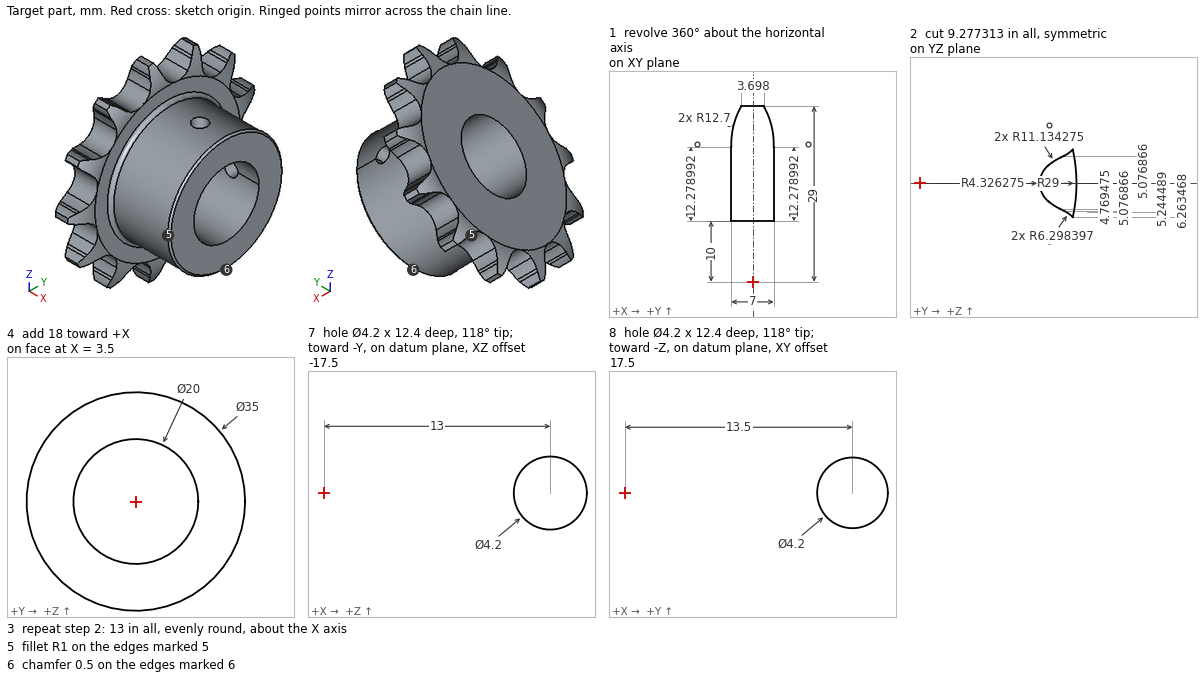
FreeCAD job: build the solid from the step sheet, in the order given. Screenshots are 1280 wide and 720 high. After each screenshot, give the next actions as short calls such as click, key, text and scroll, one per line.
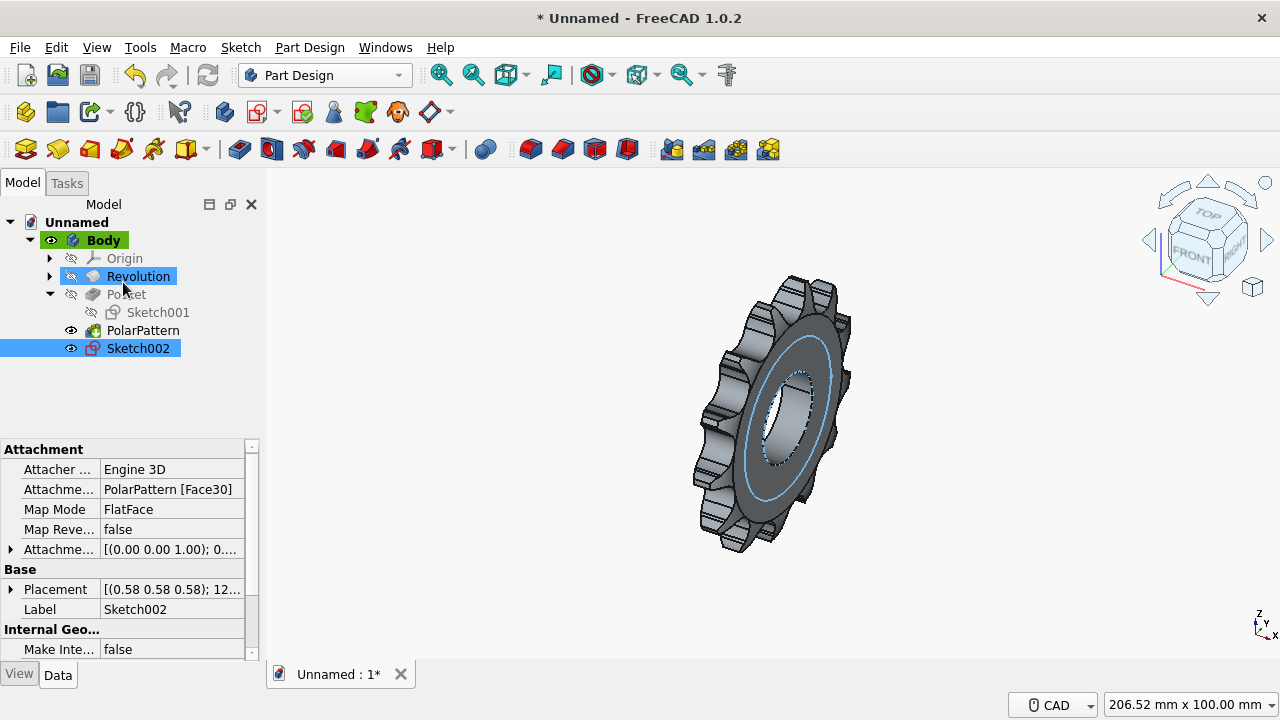
click(26, 150)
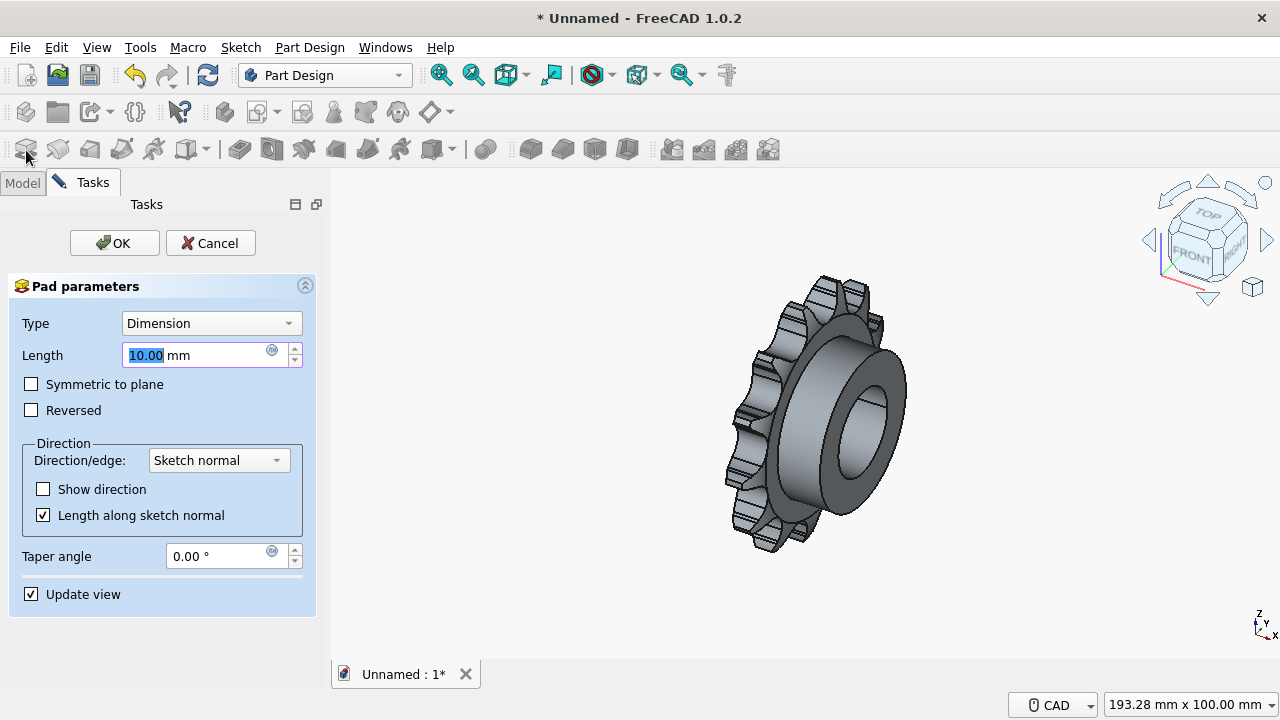
text(18)
key(Tab)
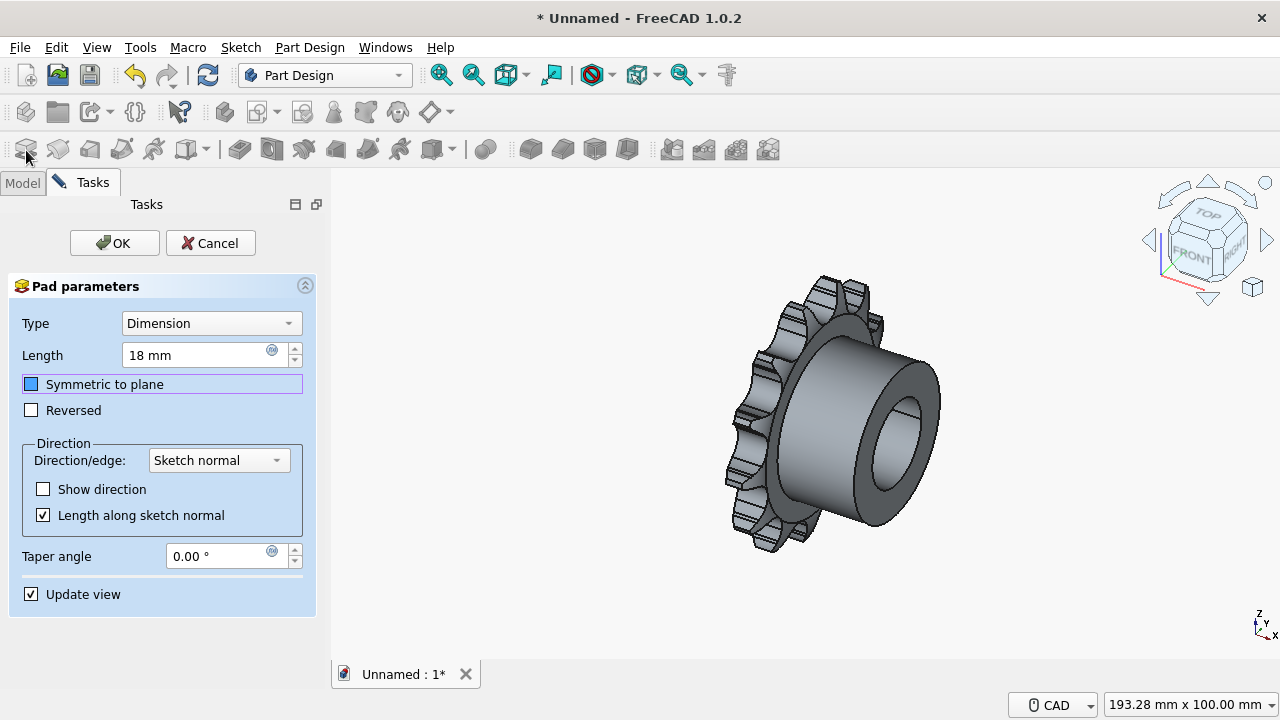
click(115, 243)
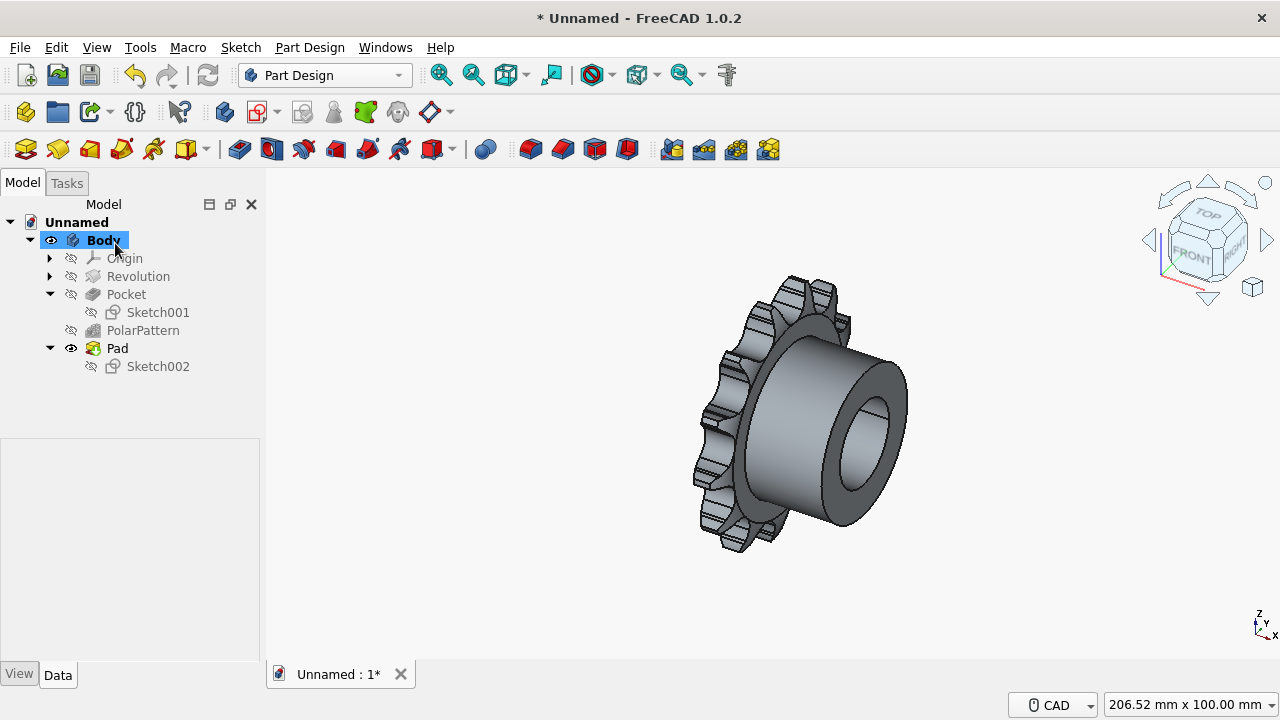
key(0)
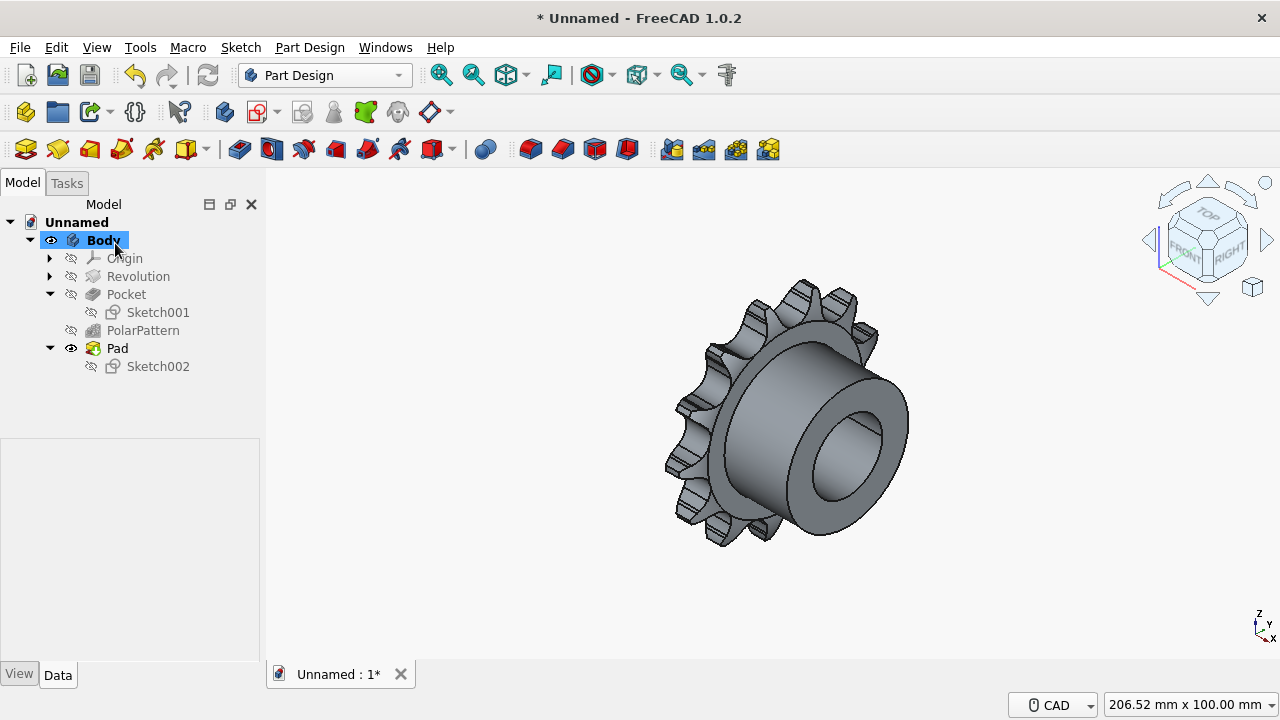
key(2)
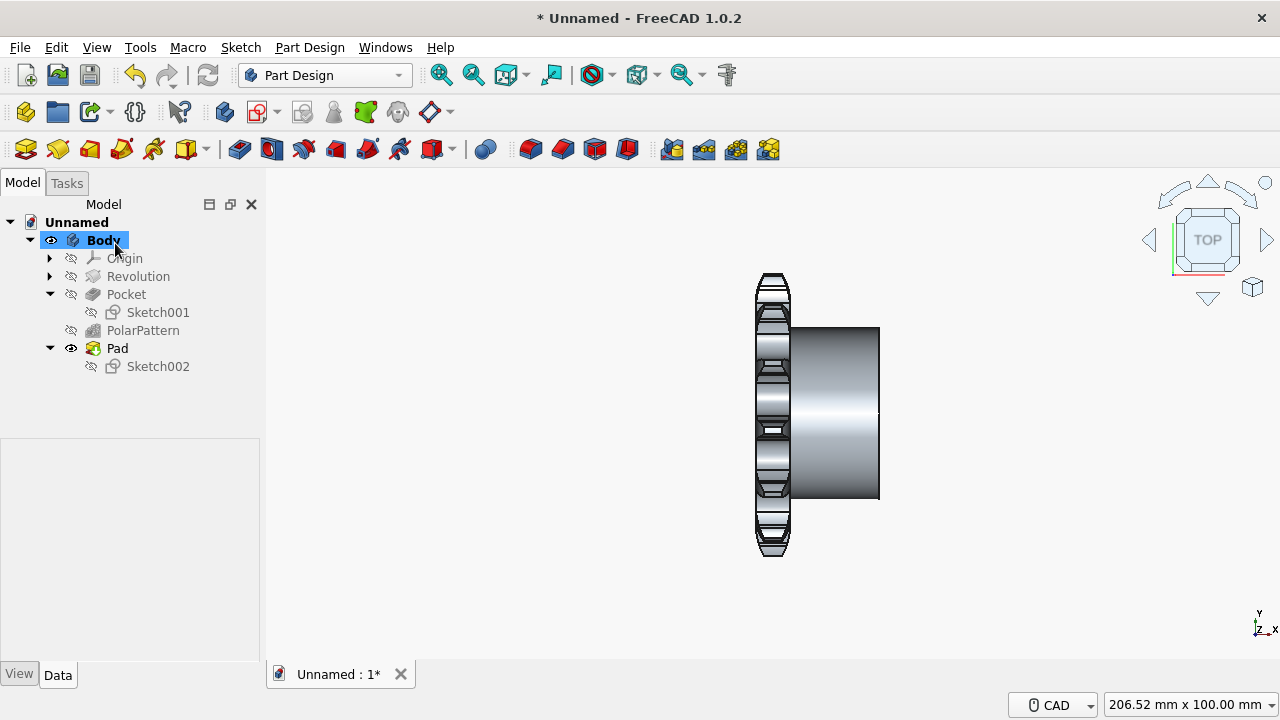
key(1)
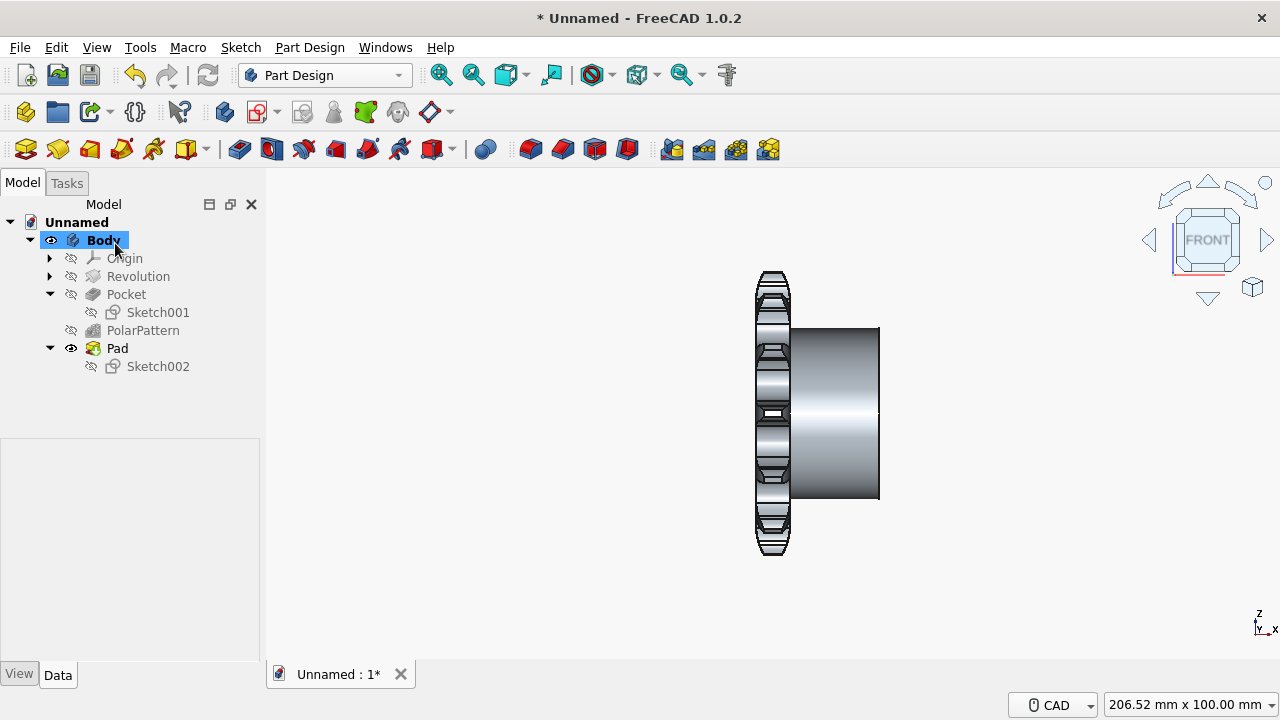
key(3)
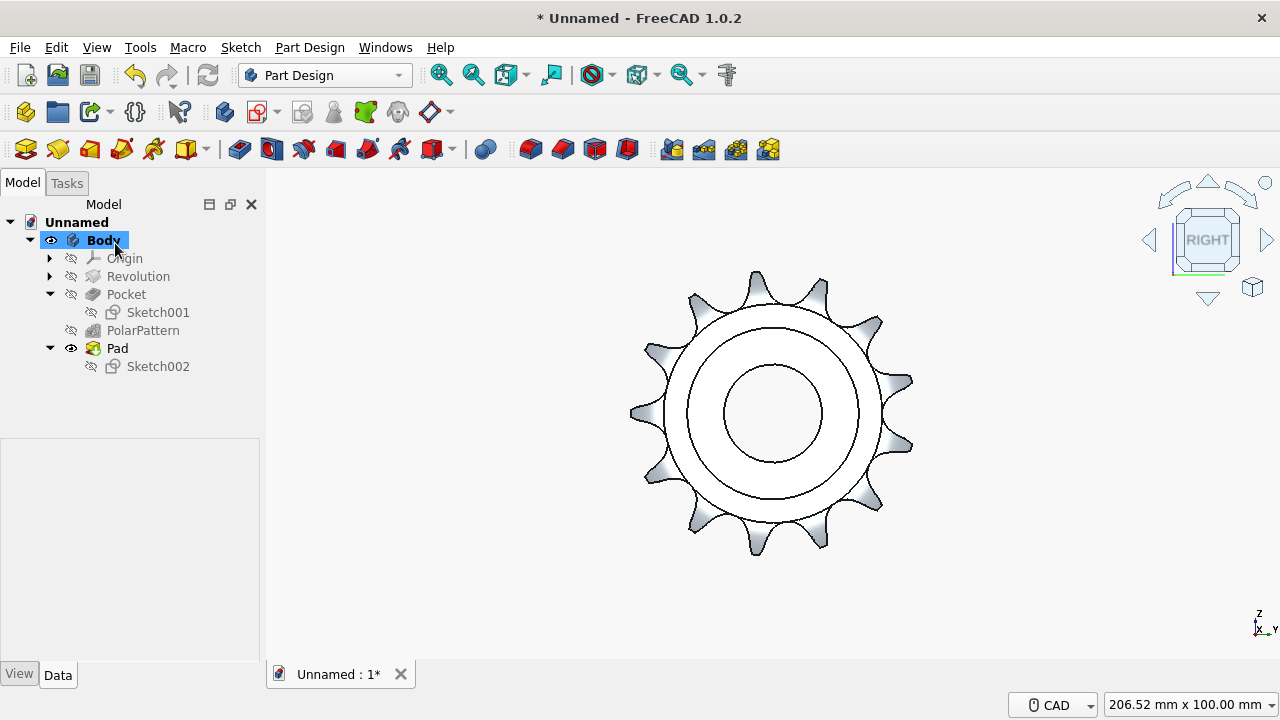
key(5)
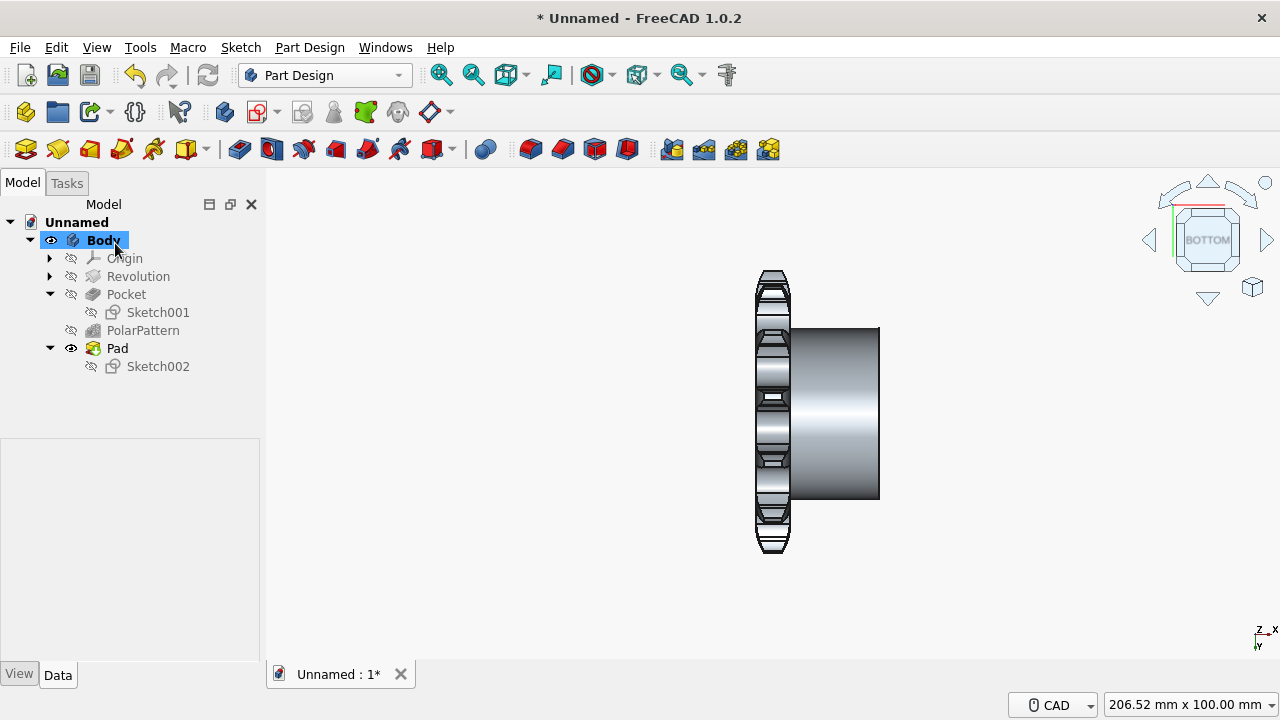
key(4)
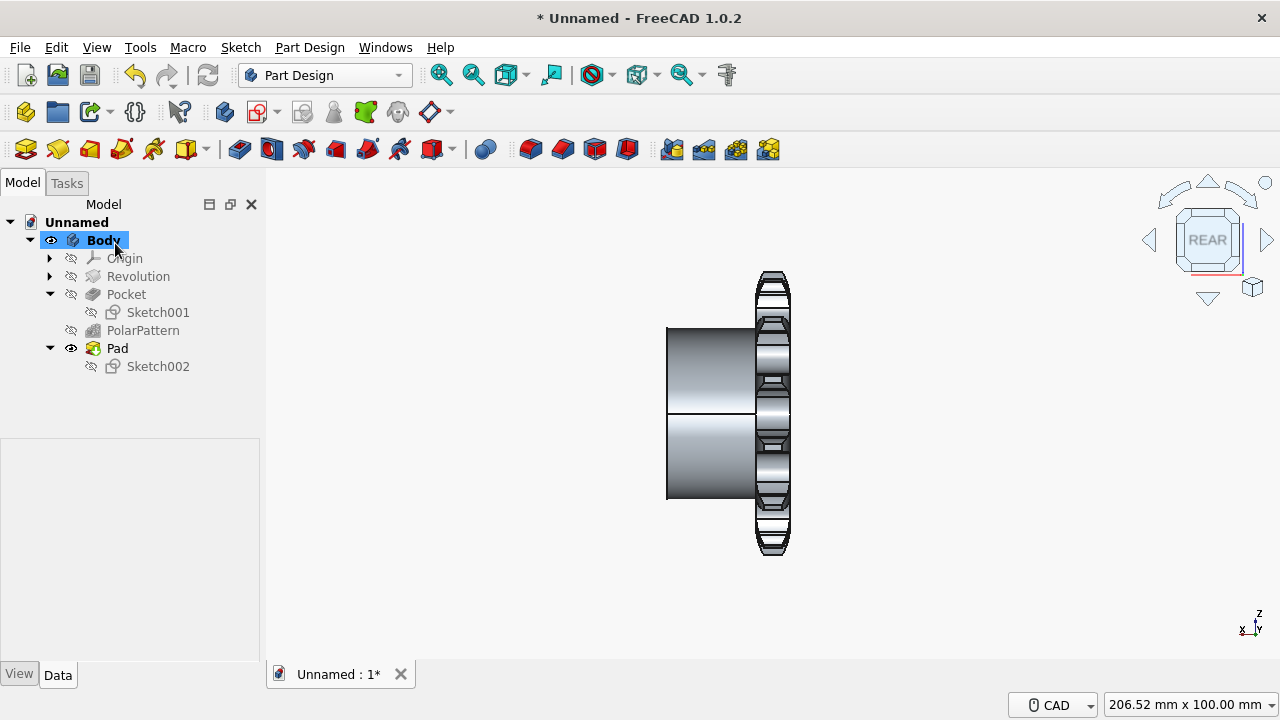
key(6)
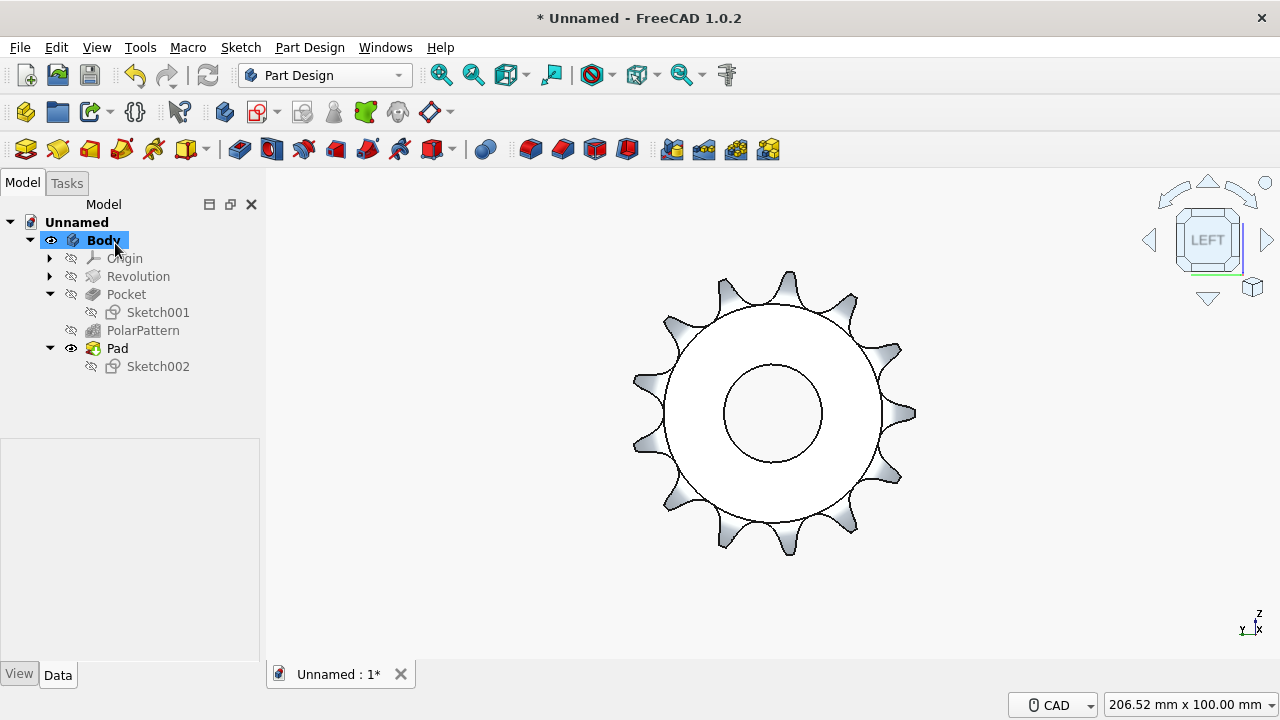
key(v)
key(3)